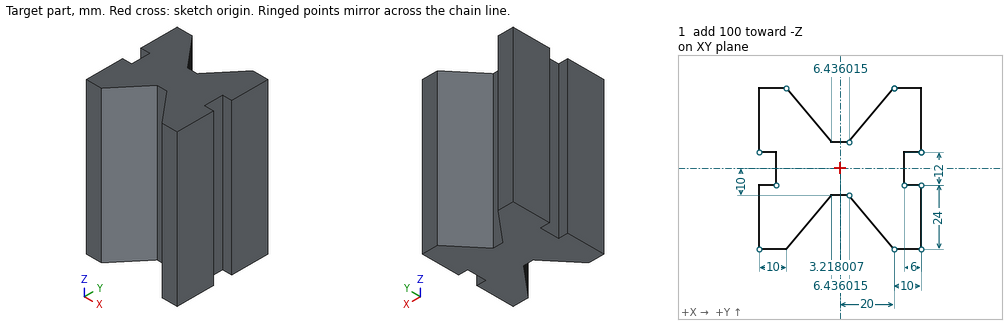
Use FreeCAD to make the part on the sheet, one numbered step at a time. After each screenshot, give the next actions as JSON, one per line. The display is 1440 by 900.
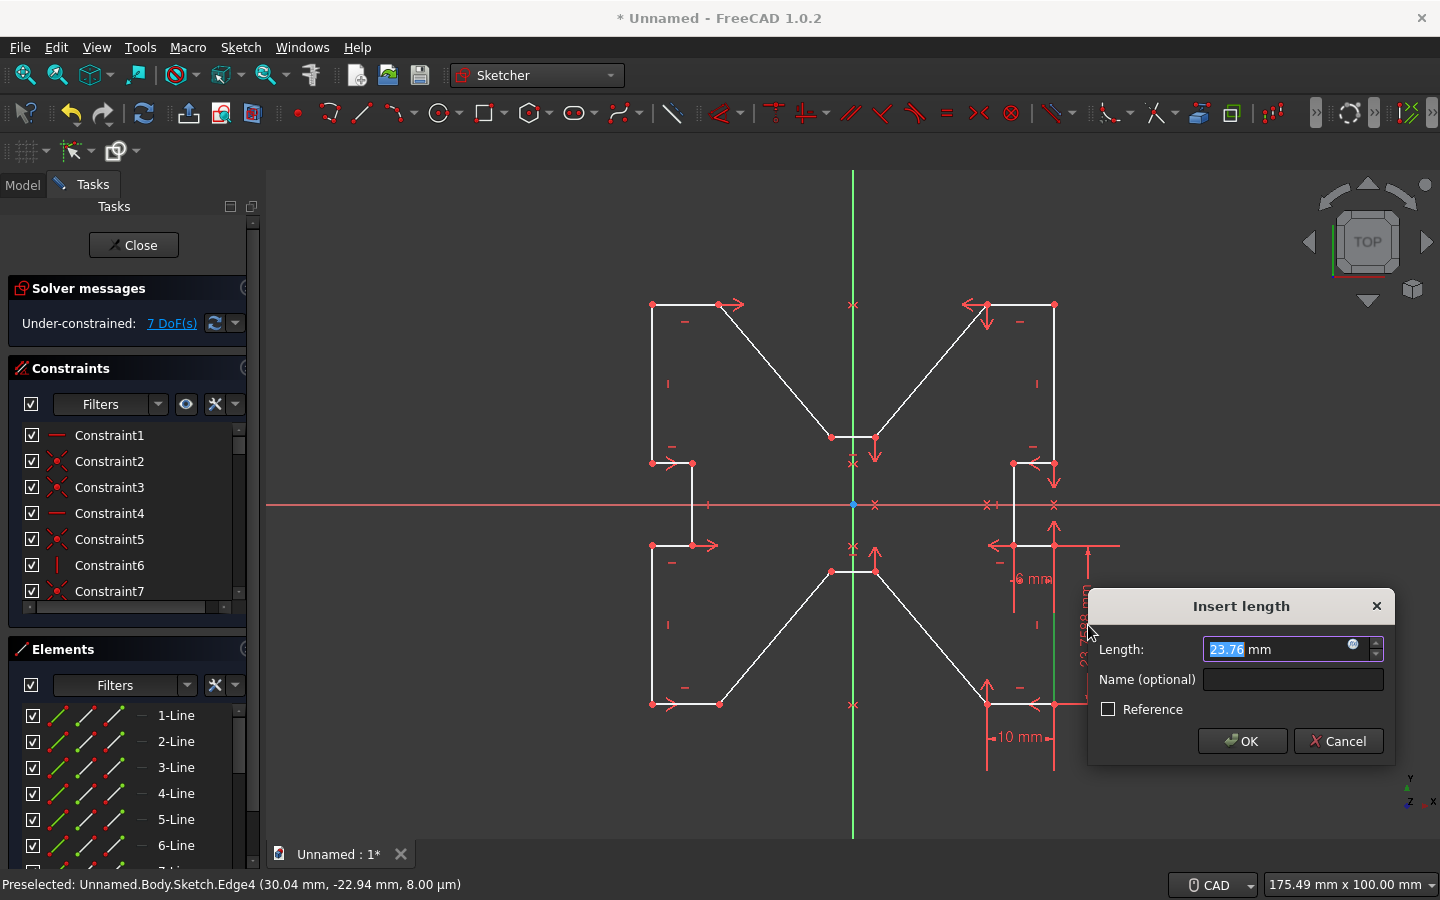
{"action": "type", "text": "24"}
{"action": "key", "text": "Return"}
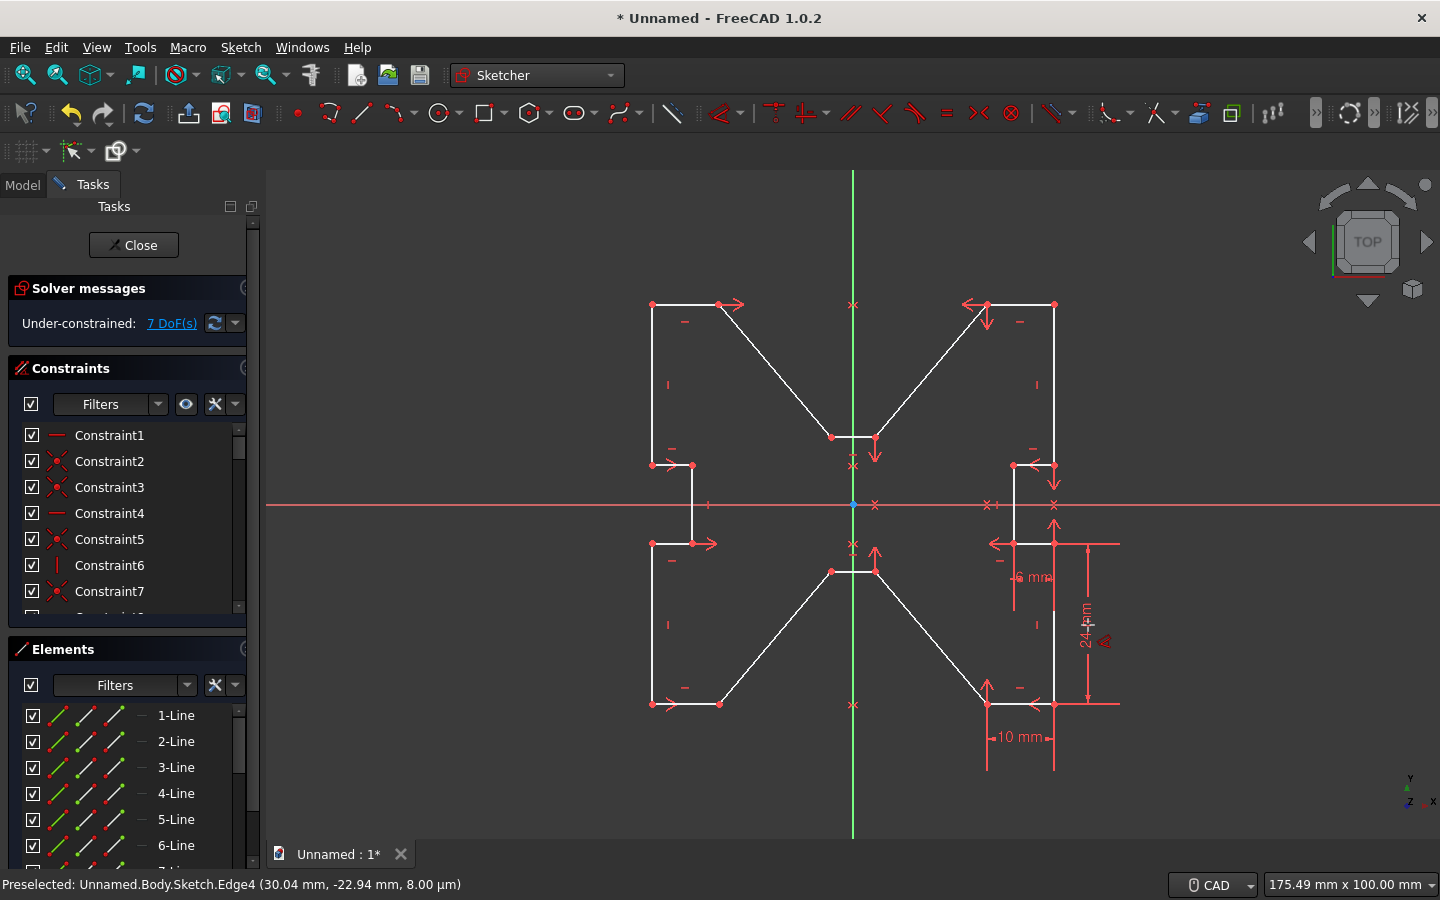
{"action": "left_click", "coordinate": [1014, 520]}
{"action": "left_click", "coordinate": [1048, 486]}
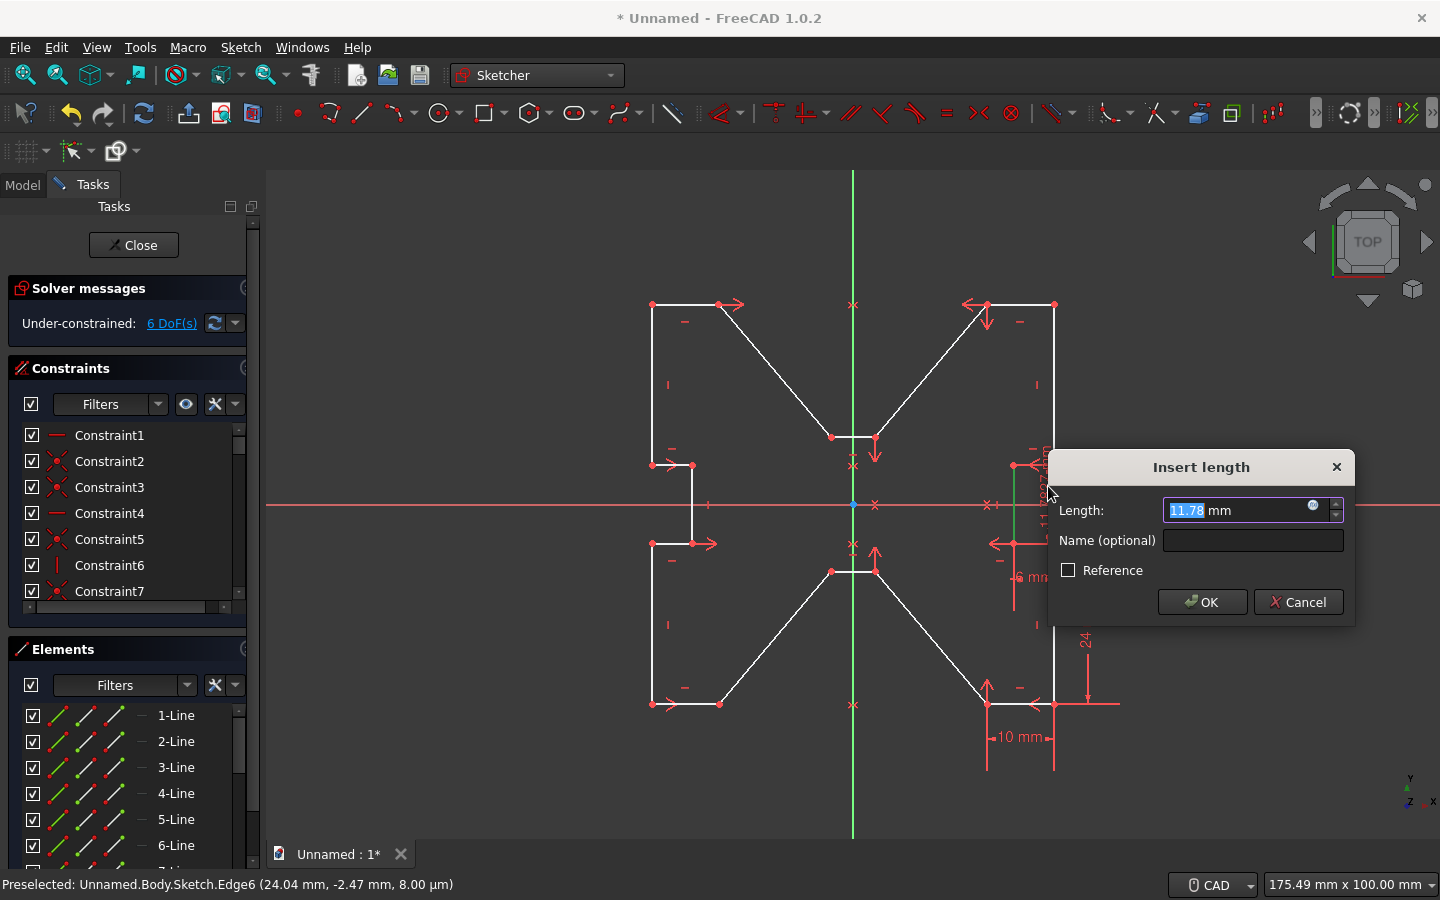
{"action": "type", "text": "12"}
{"action": "key", "text": "Return"}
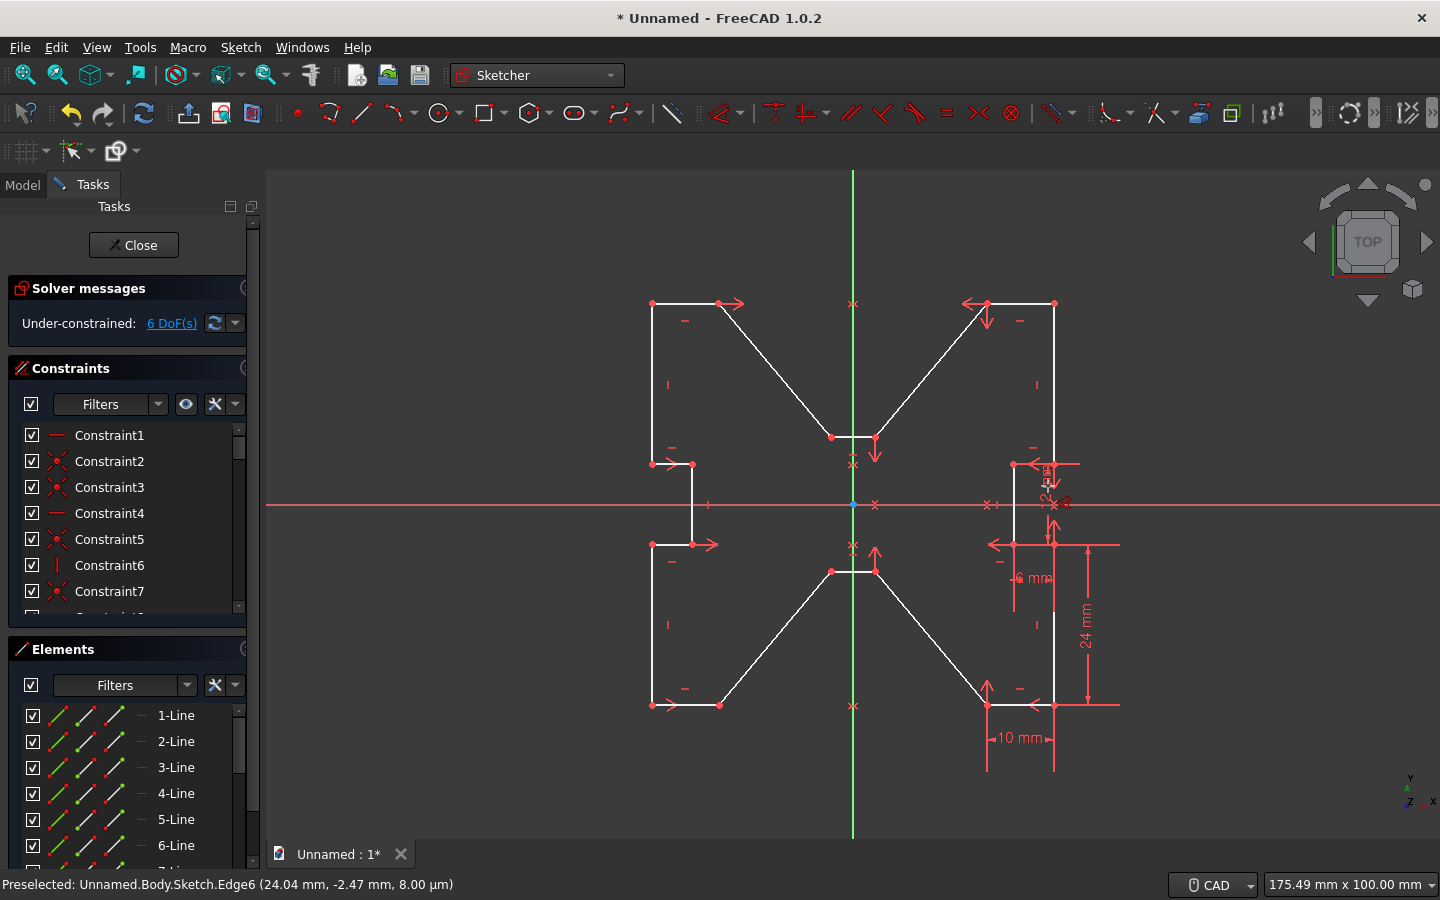
{"action": "left_click", "coordinate": [672, 705]}
{"action": "left_click", "coordinate": [686, 739]}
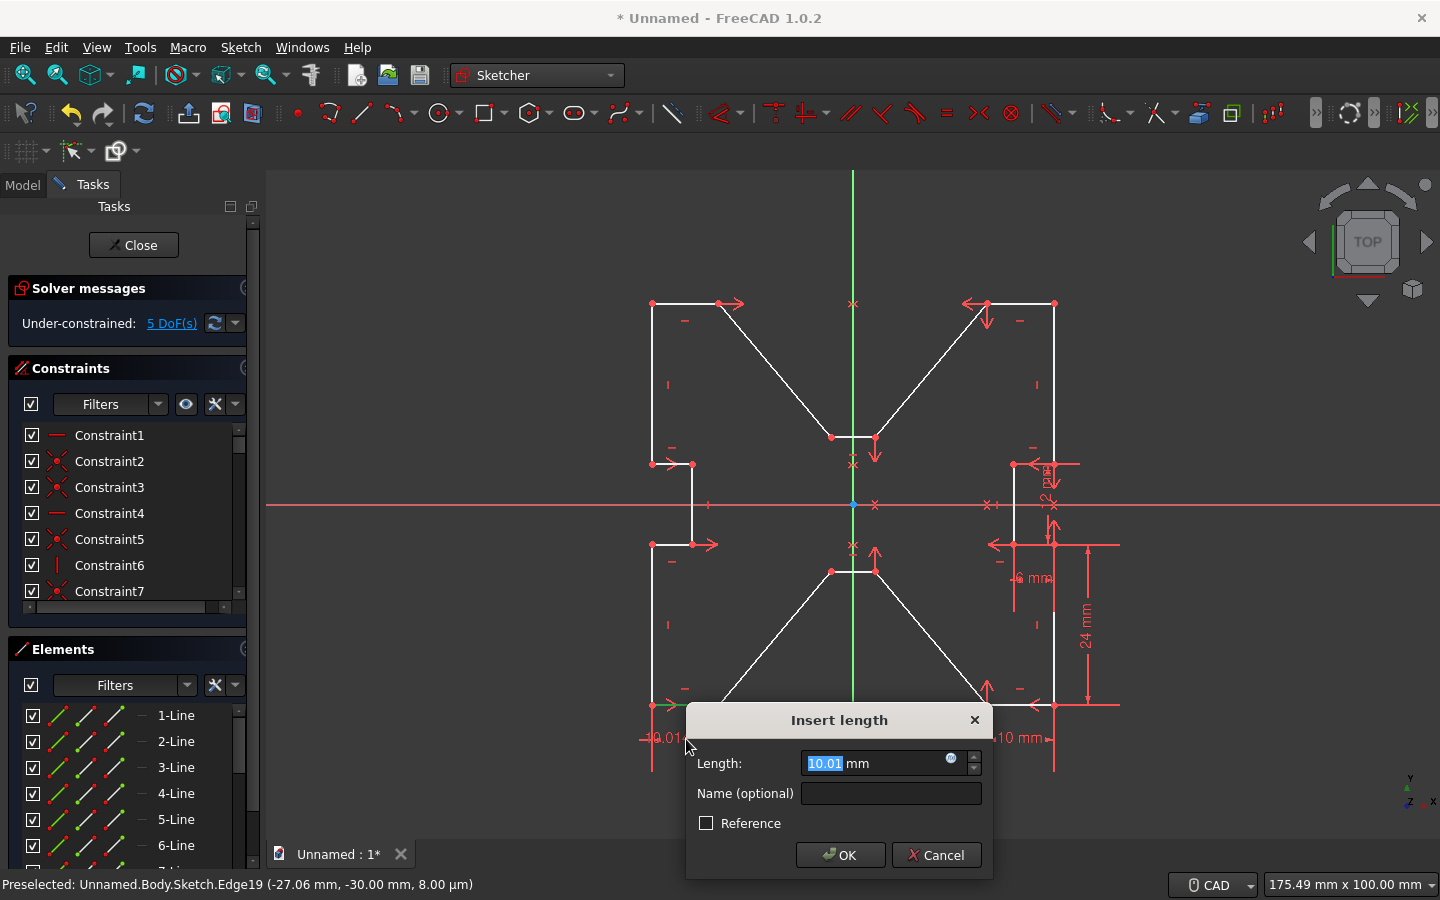
{"action": "type", "text": "10"}
{"action": "key", "text": "Return"}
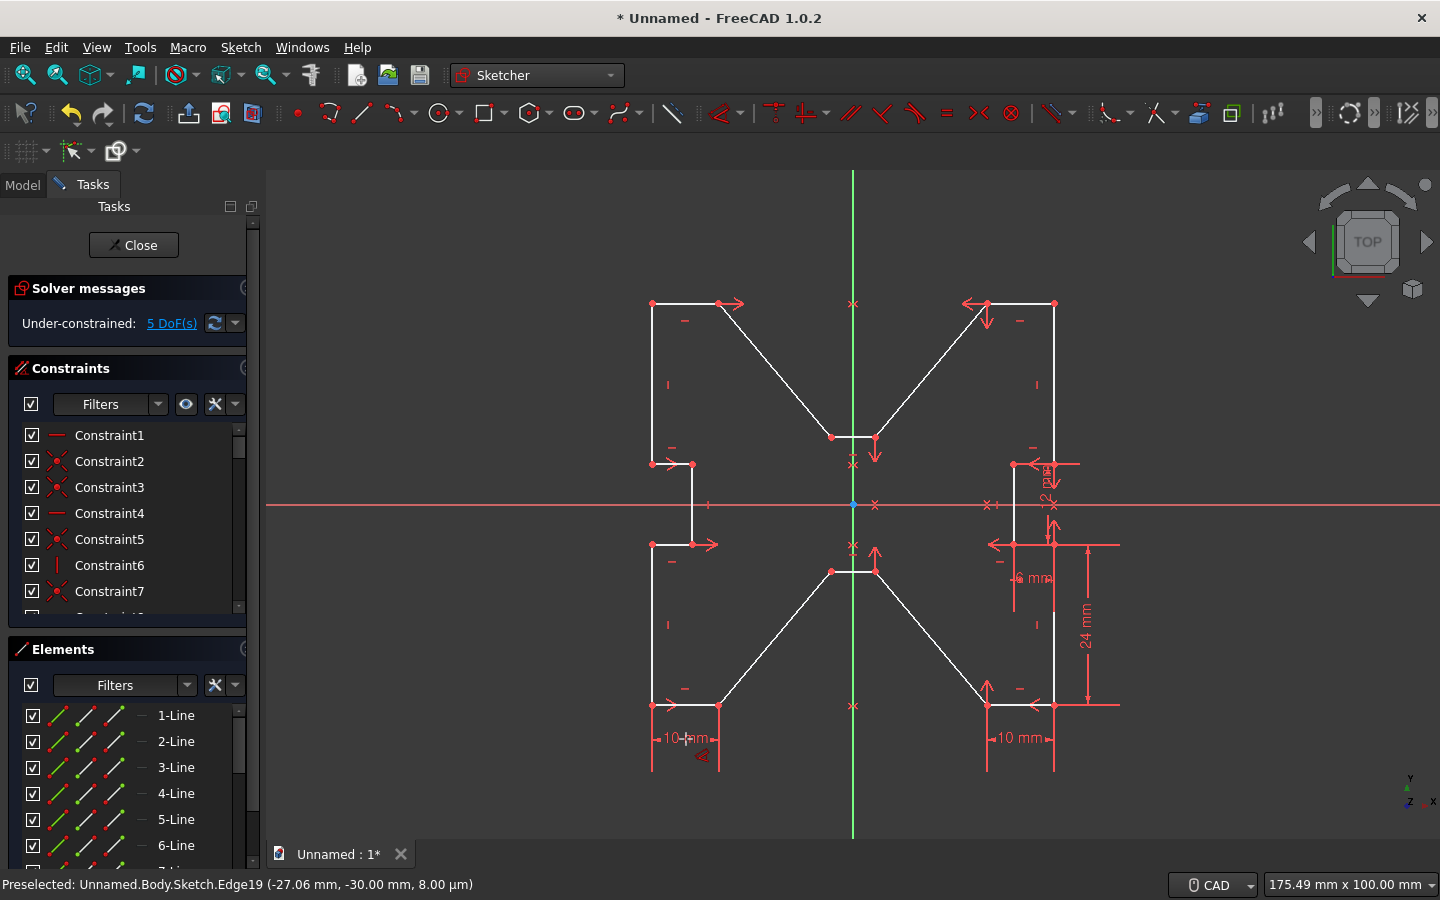
{"action": "left_click", "coordinate": [831, 572]}
{"action": "left_click", "coordinate": [797, 538]}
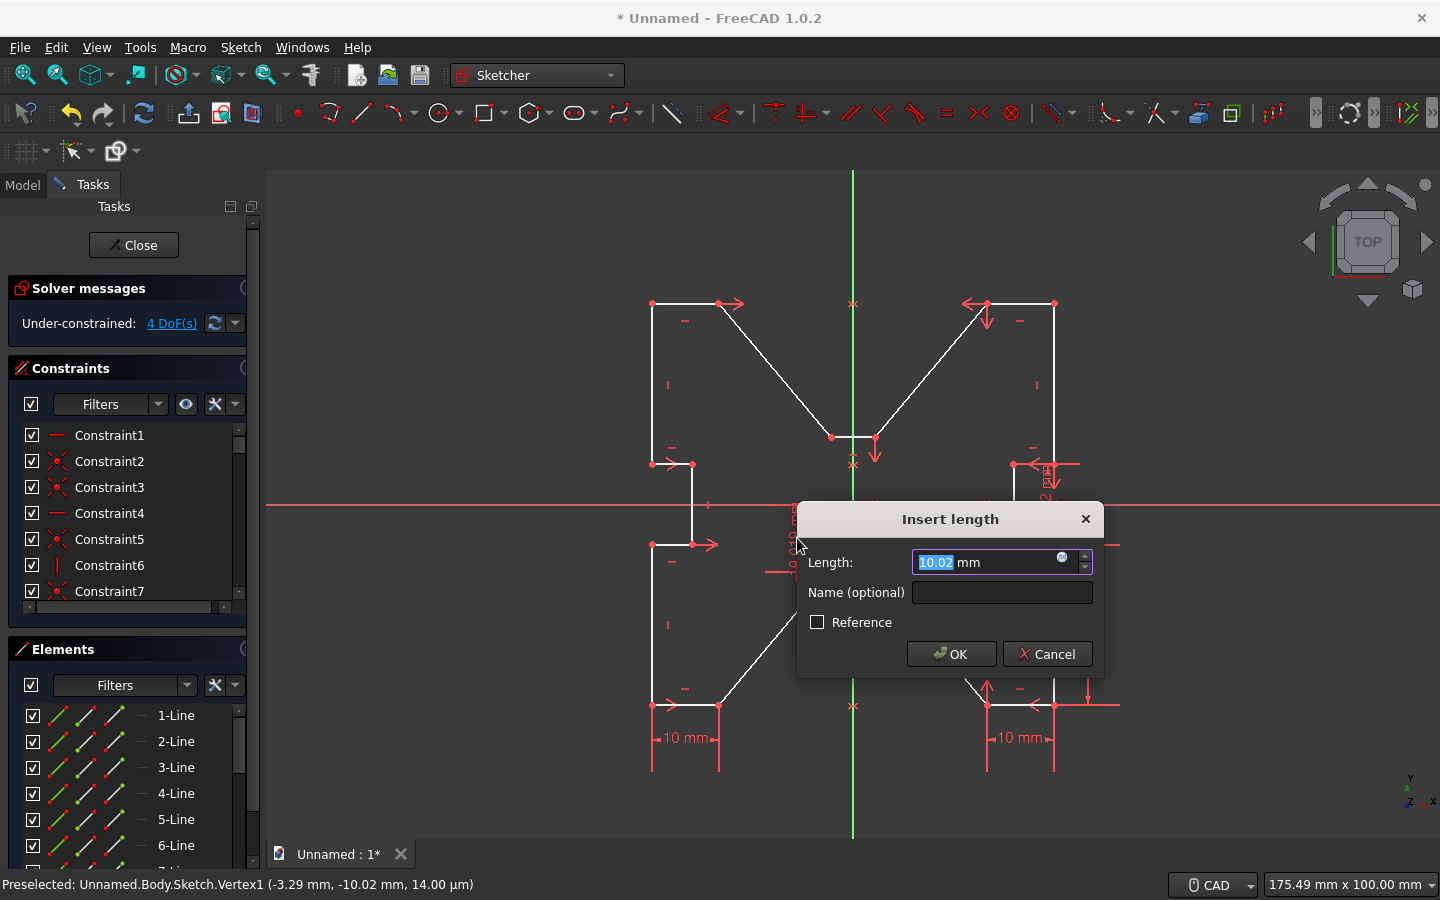
{"action": "type", "text": "10"}
{"action": "key", "text": "Return"}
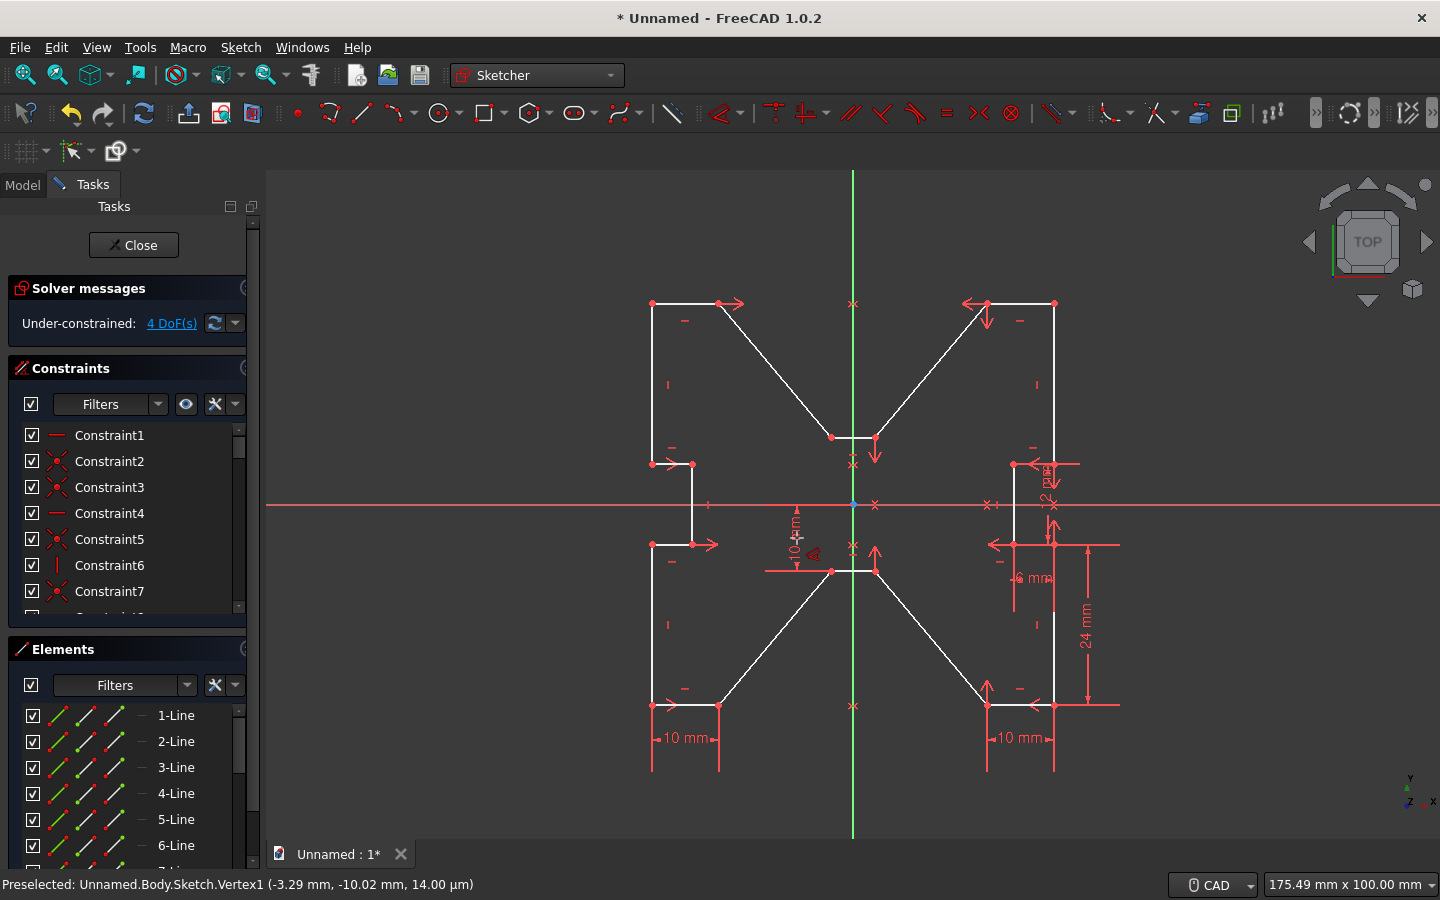
{"action": "left_click", "coordinate": [987, 705]}
{"action": "left_click", "coordinate": [920, 739]}